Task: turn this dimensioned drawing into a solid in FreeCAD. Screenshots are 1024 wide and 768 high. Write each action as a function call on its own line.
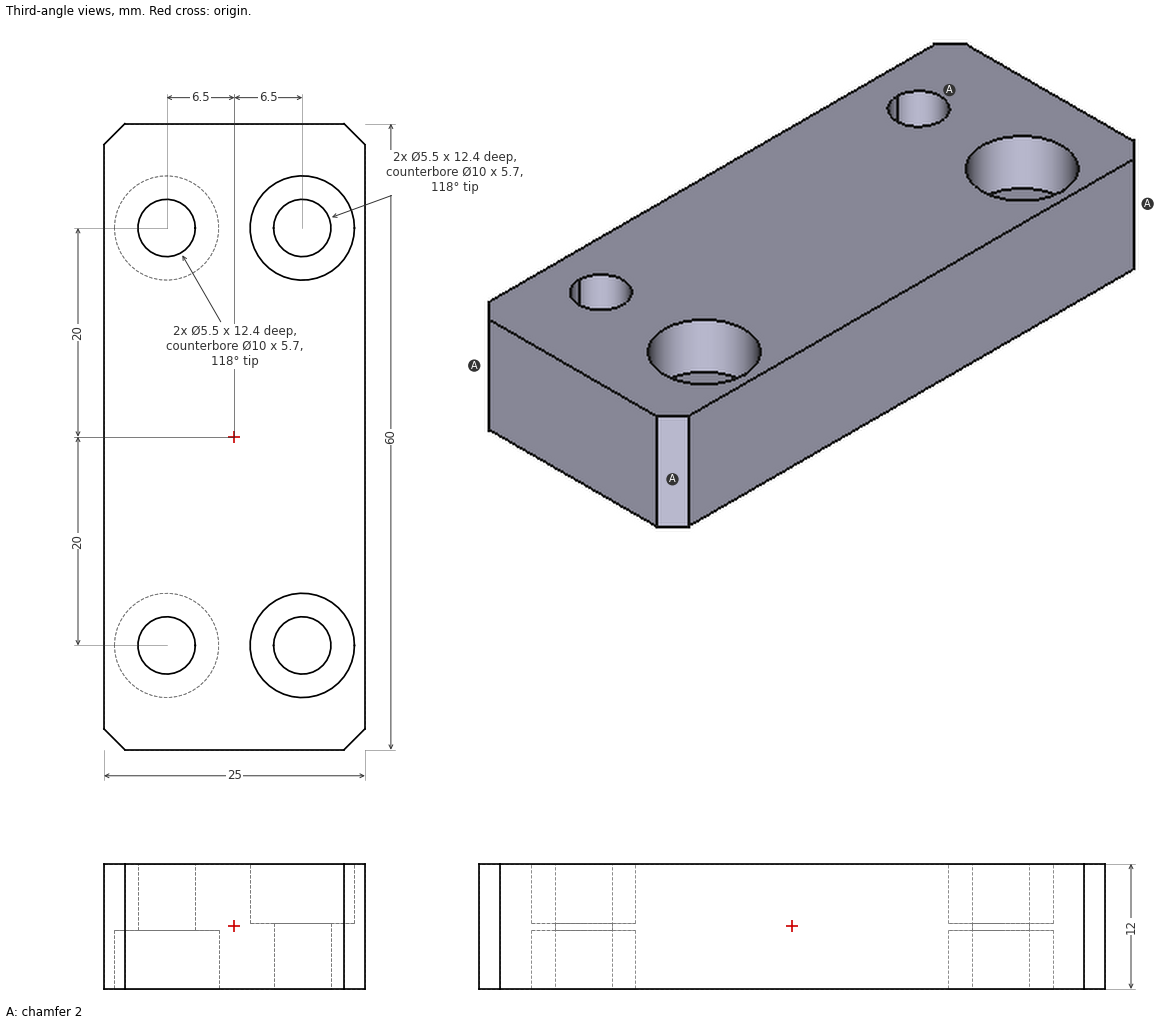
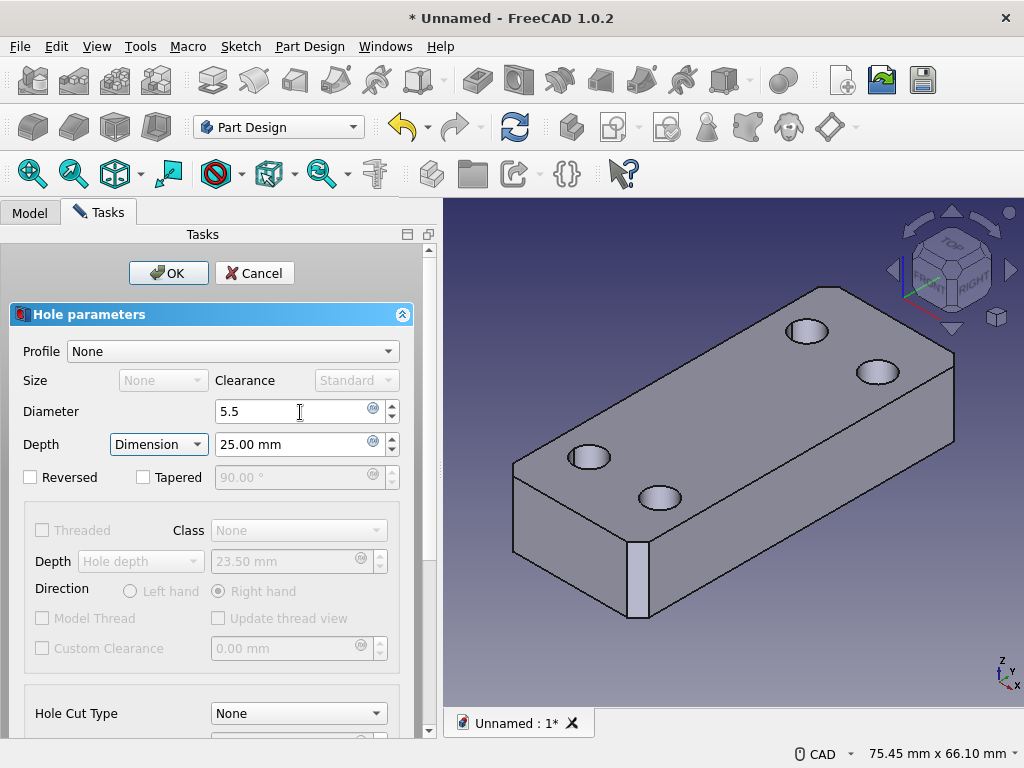
triple_click(300, 444)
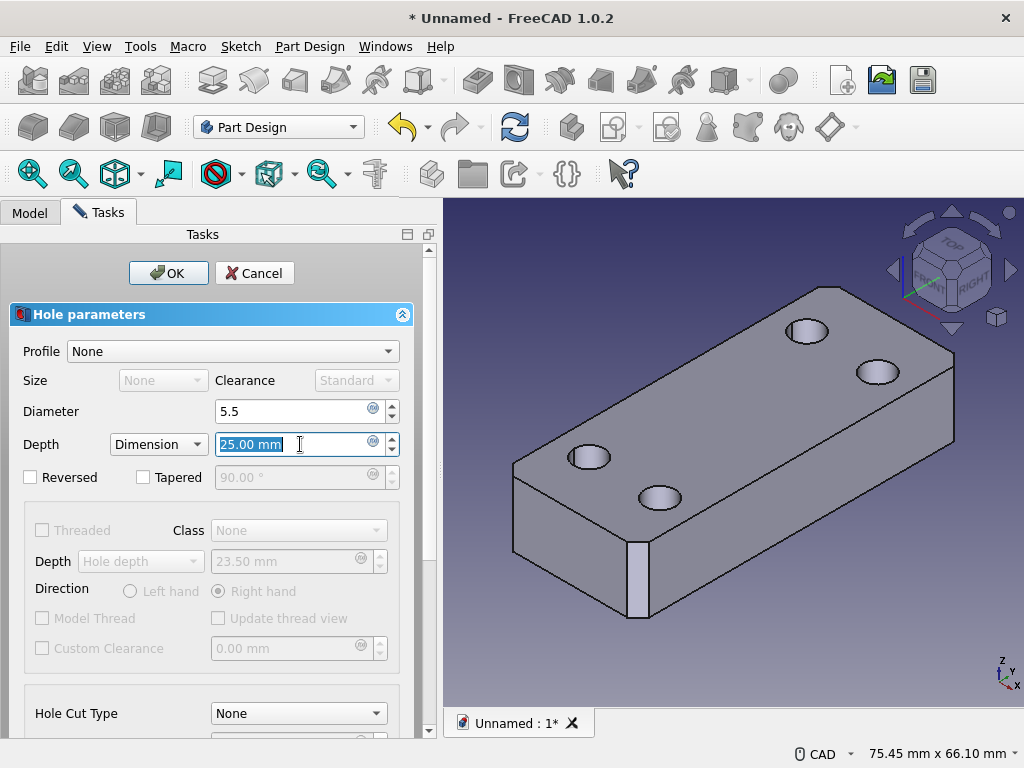
text(12.4)
key(Tab)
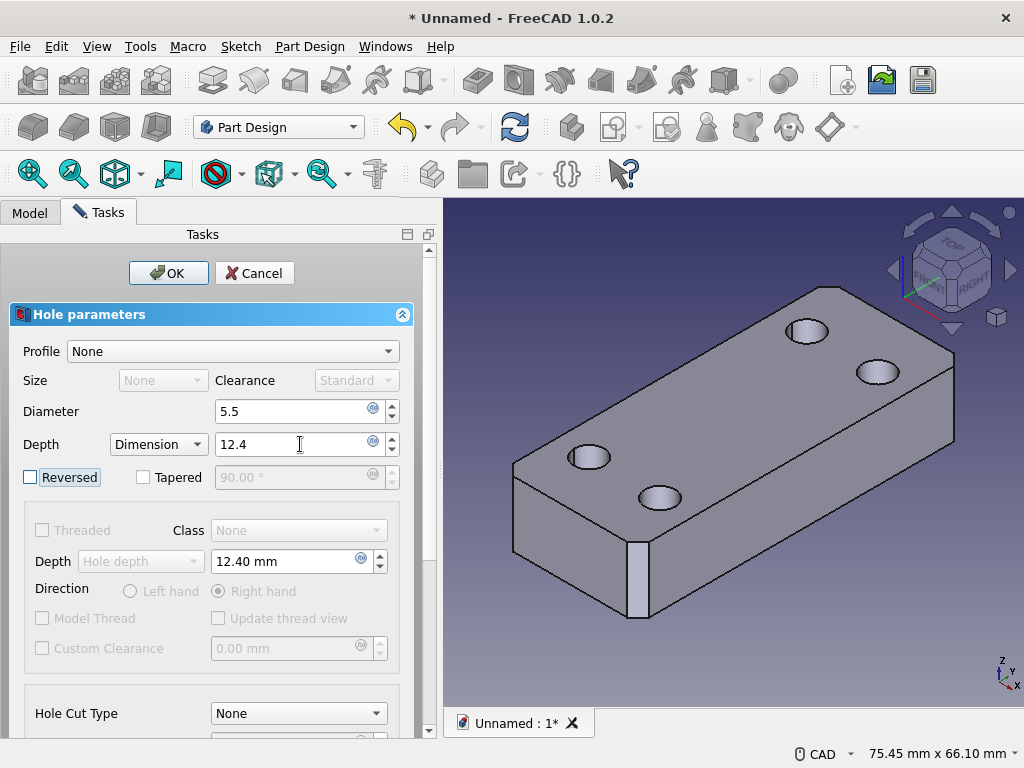
click(300, 714)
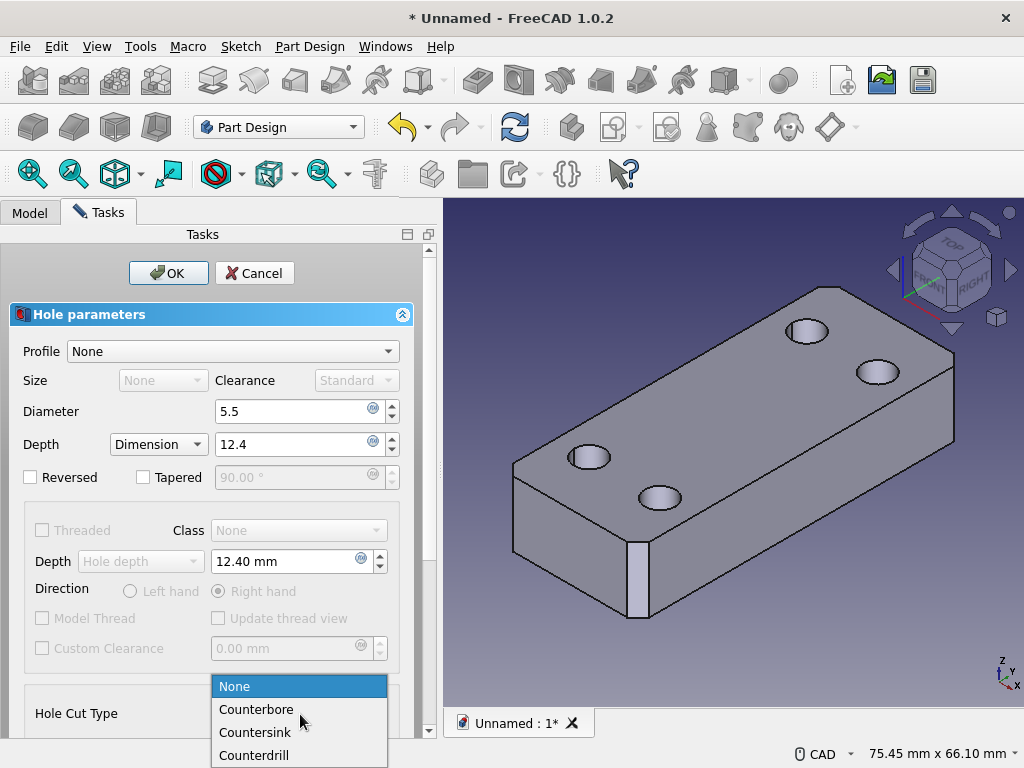
click(298, 710)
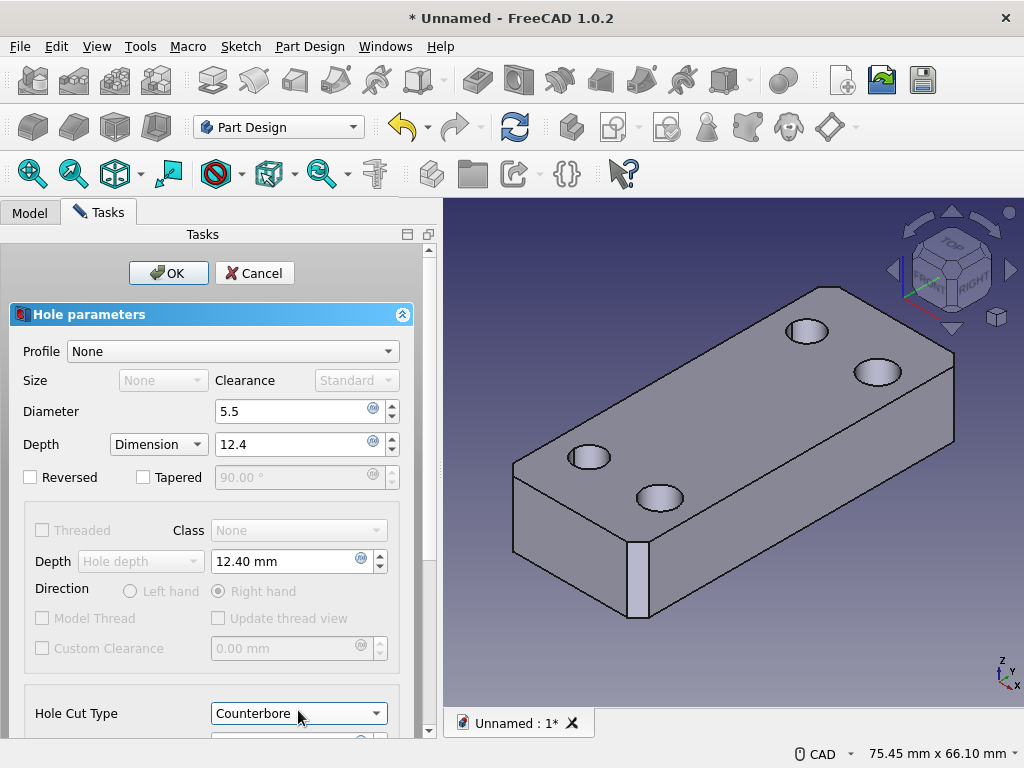
scroll(429, 491, down, 2)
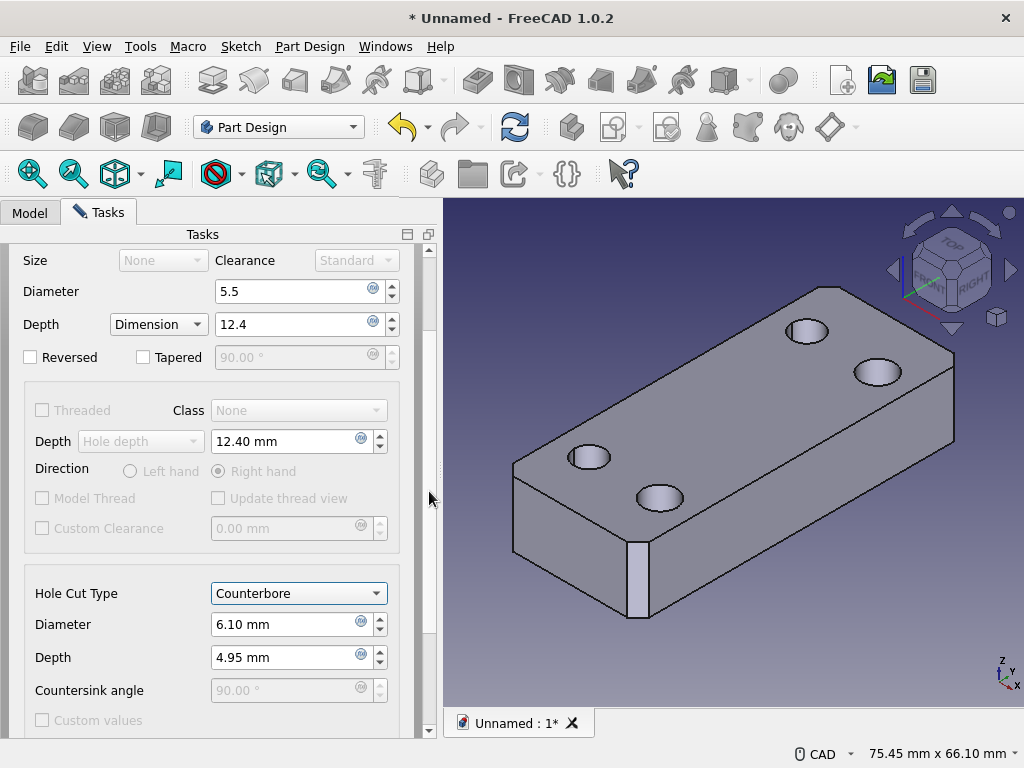
triple_click(292, 624)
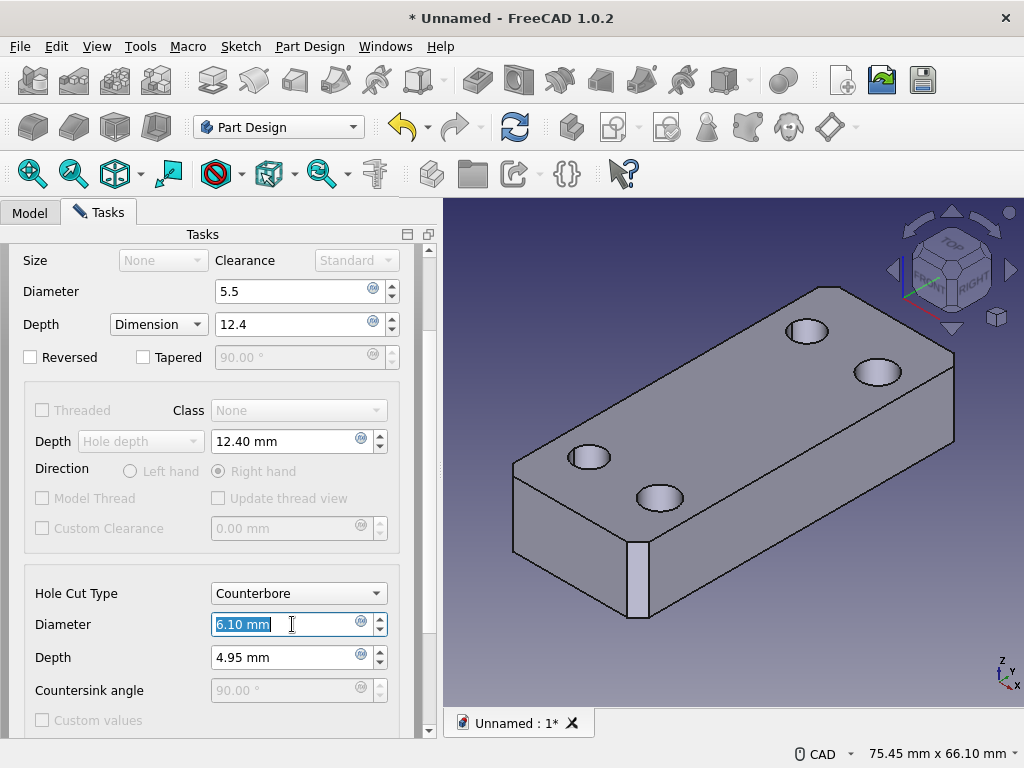
text(10)
key(Tab)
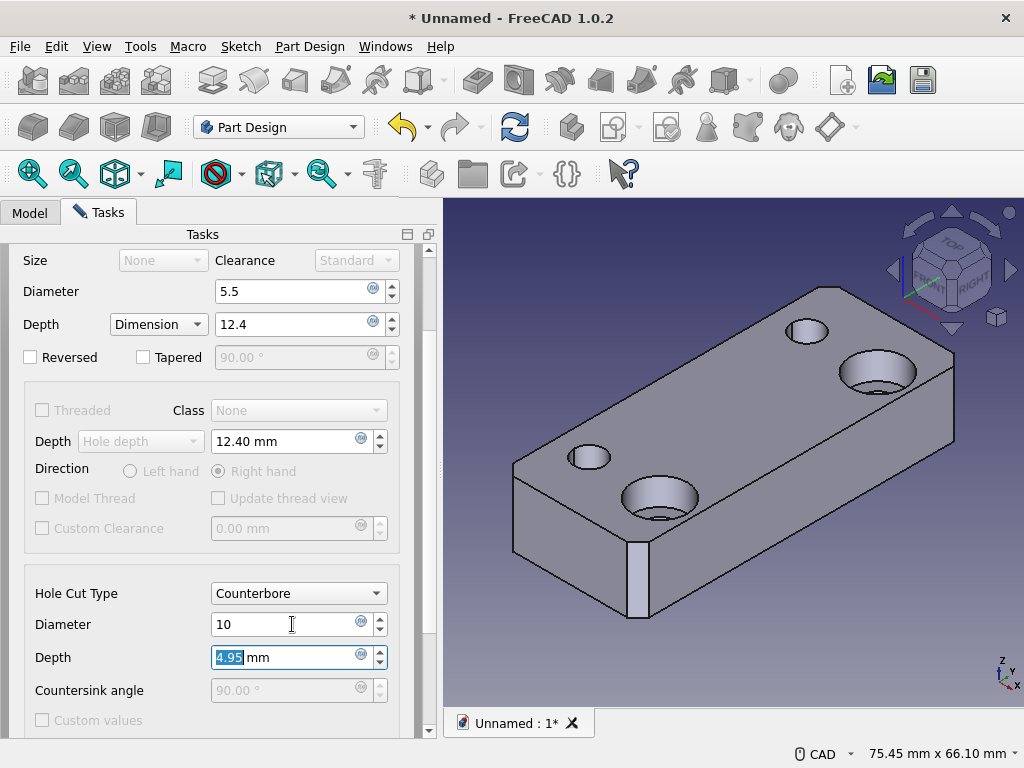
text(5.7)
key(Tab)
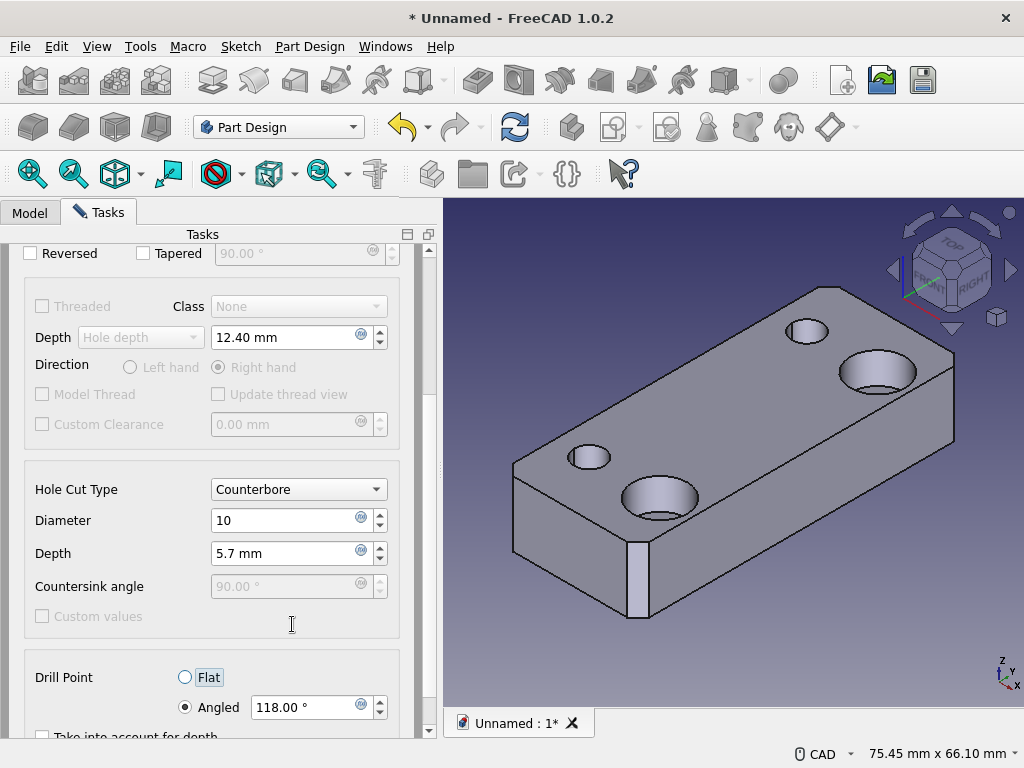
scroll(429, 491, up, 5)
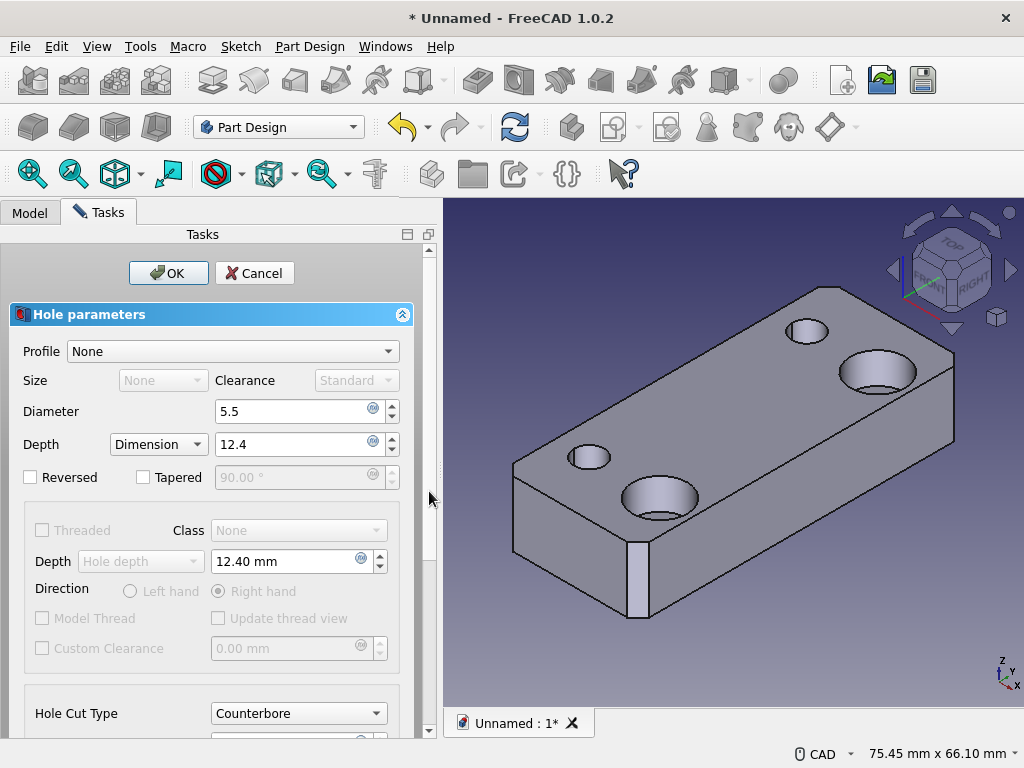
click(169, 273)